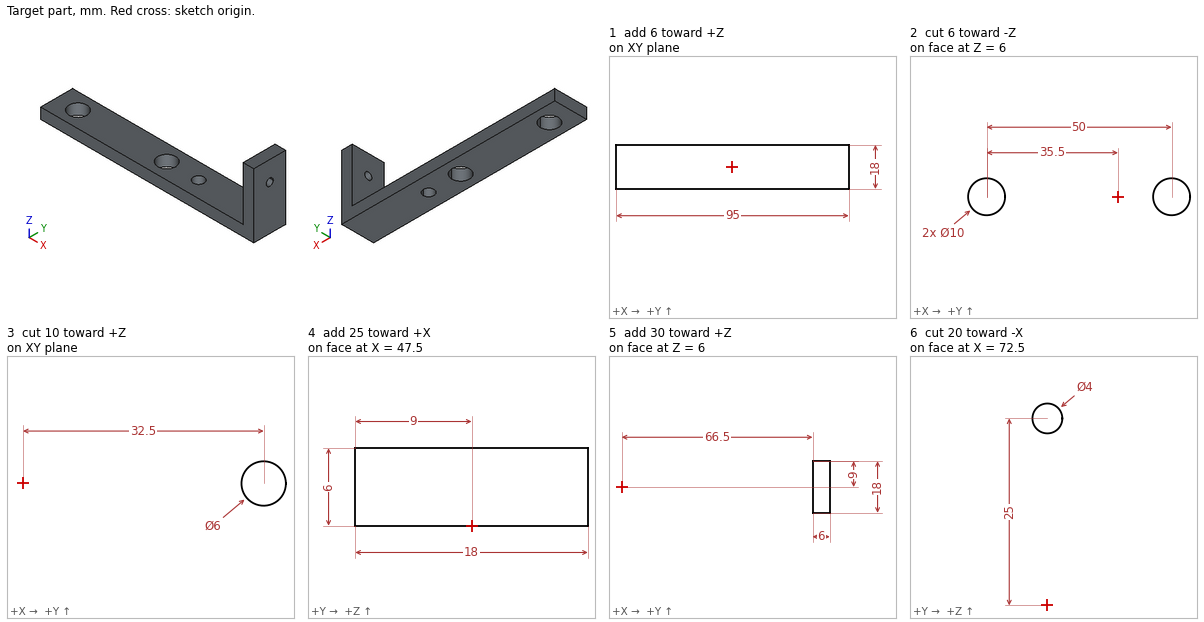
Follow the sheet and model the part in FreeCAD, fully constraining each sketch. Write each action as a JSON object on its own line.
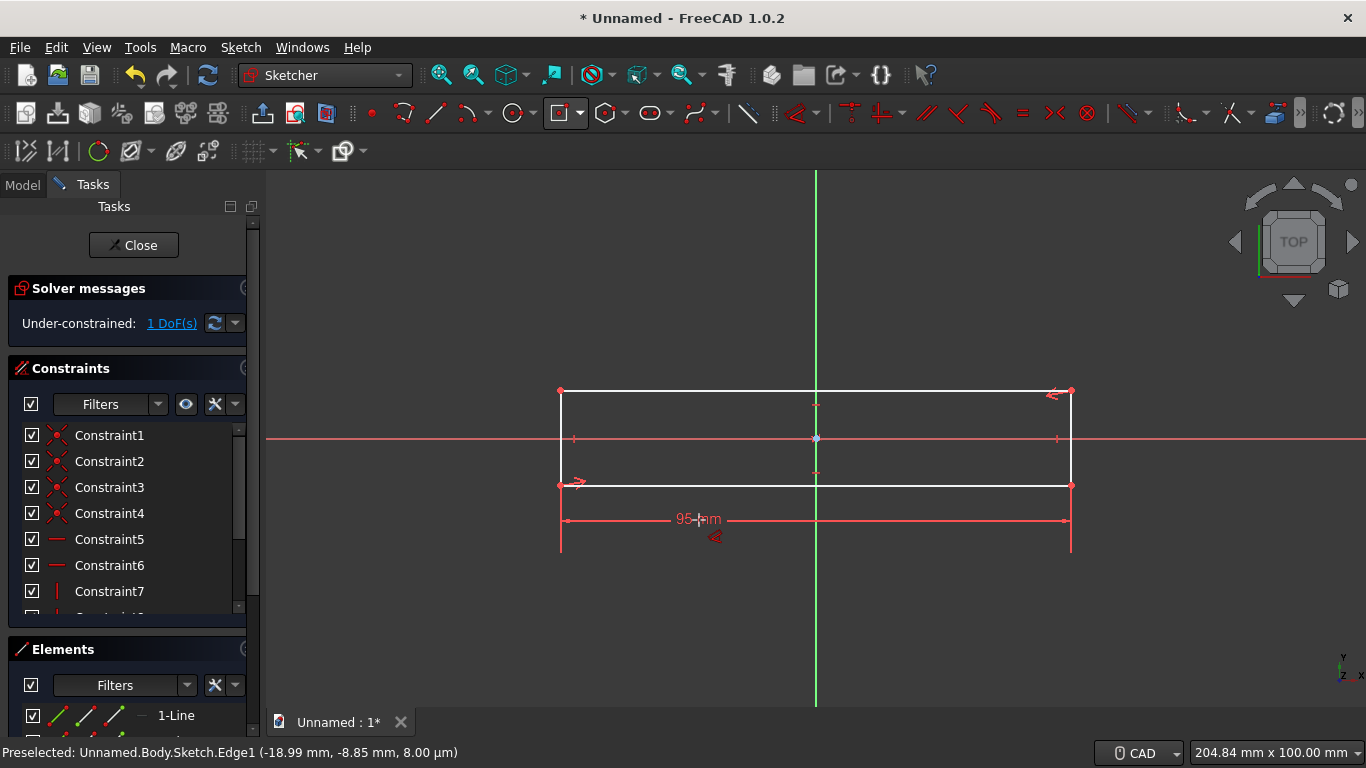
{"action": "left_click", "coordinate": [1071, 457]}
{"action": "left_click", "coordinate": [1105, 417]}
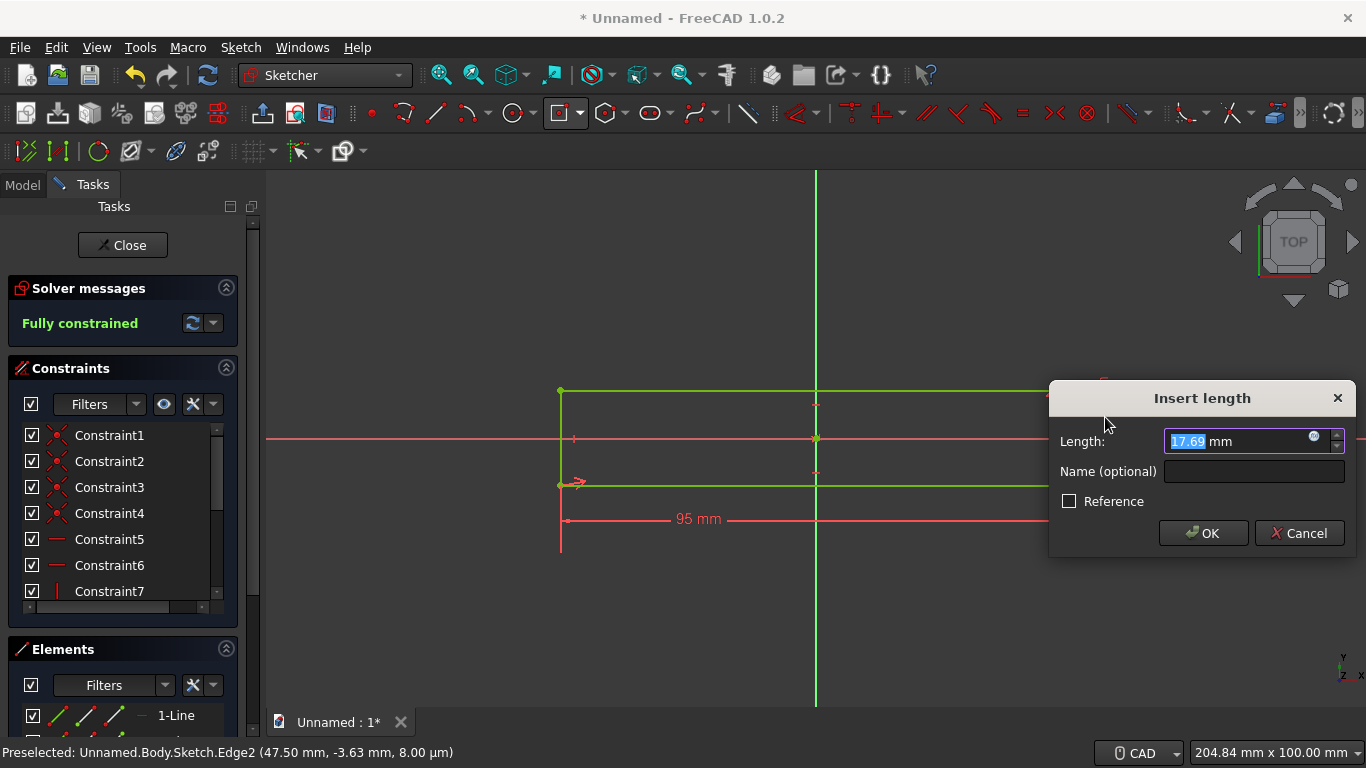
{"action": "type", "text": "18"}
{"action": "key", "text": "Return"}
{"action": "key", "text": "Escape"}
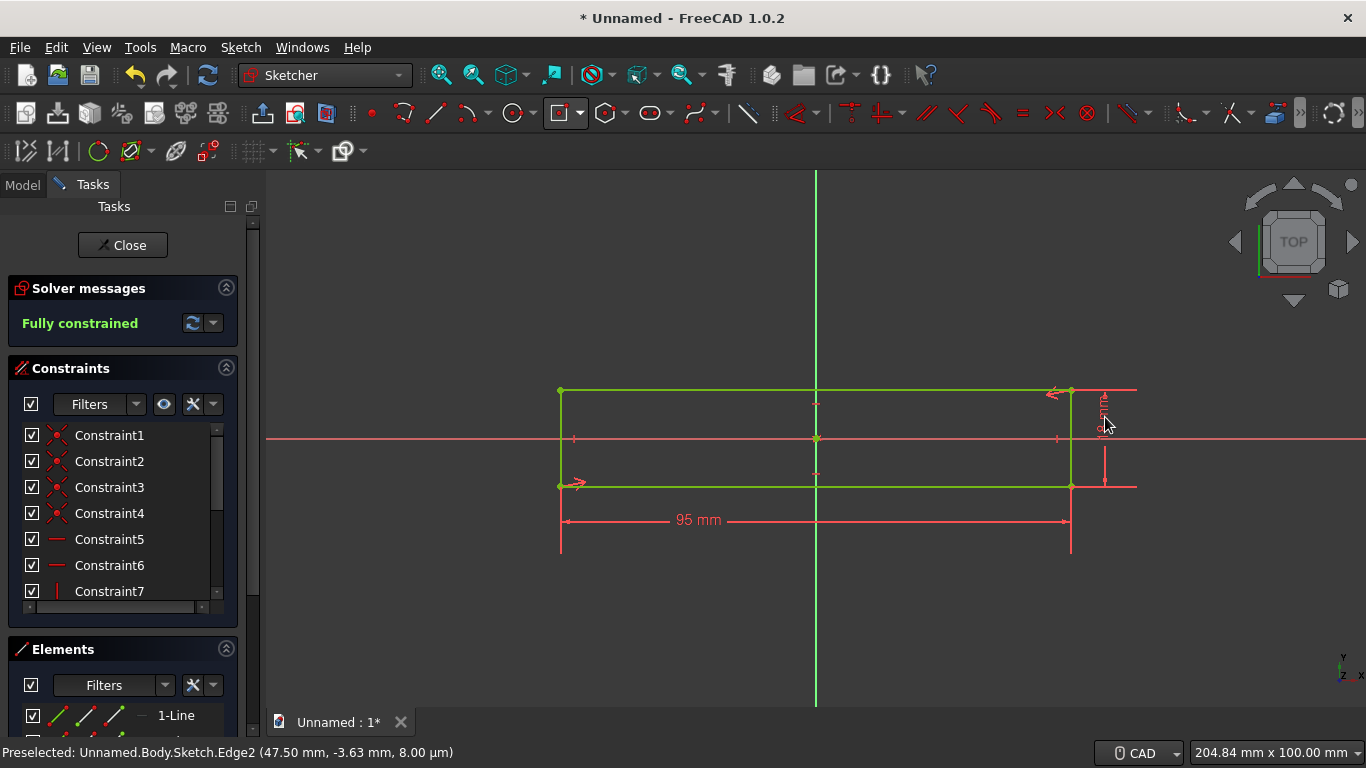
{"action": "left_click", "coordinate": [123, 245]}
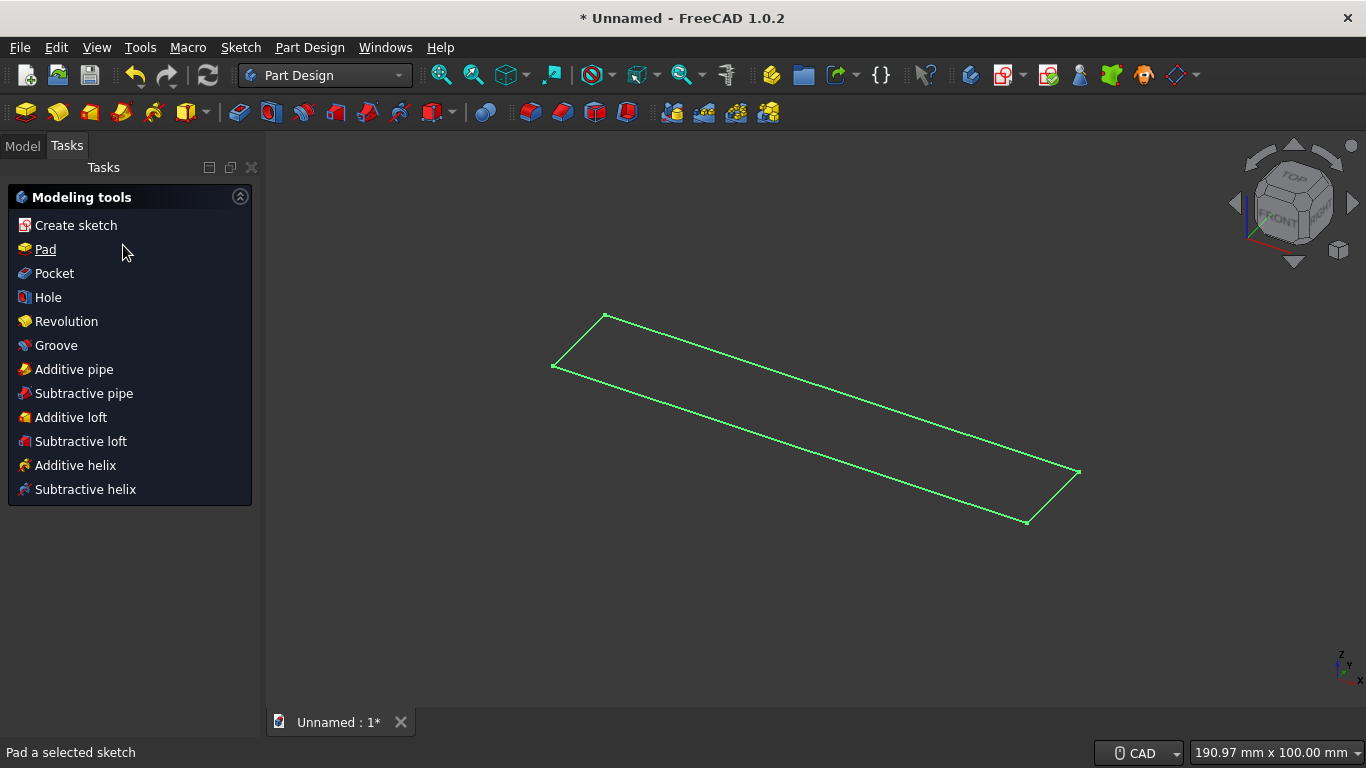
{"action": "left_click", "coordinate": [26, 112]}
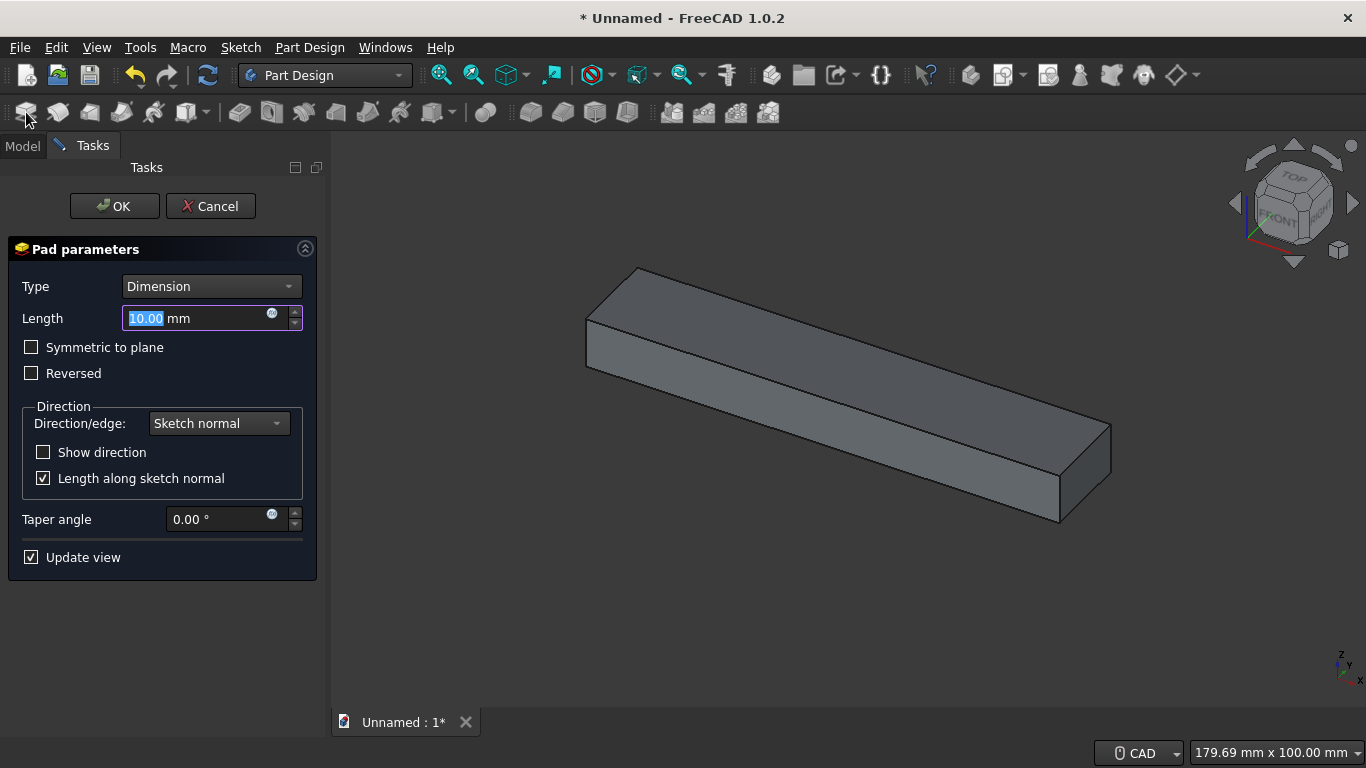
{"action": "type", "text": "6"}
{"action": "key", "text": "Tab"}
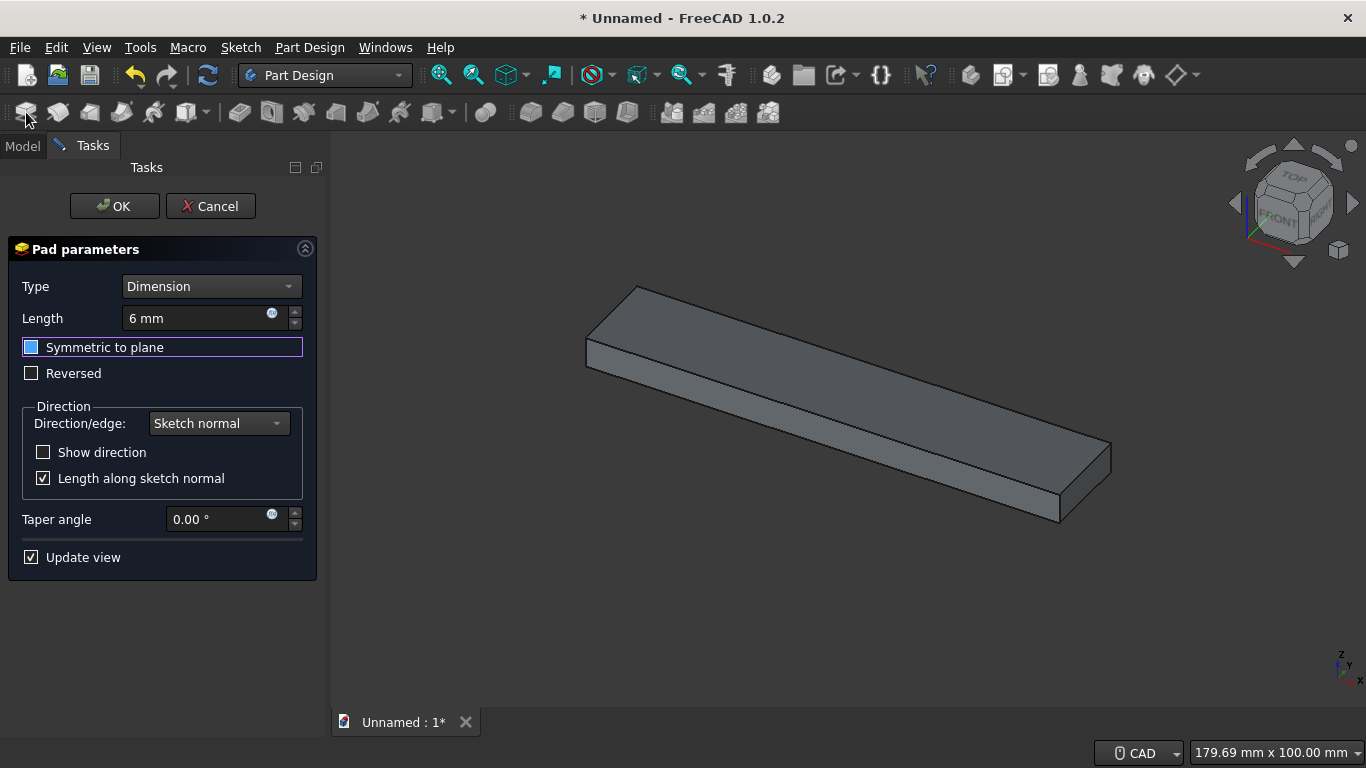
{"action": "left_click", "coordinate": [115, 206]}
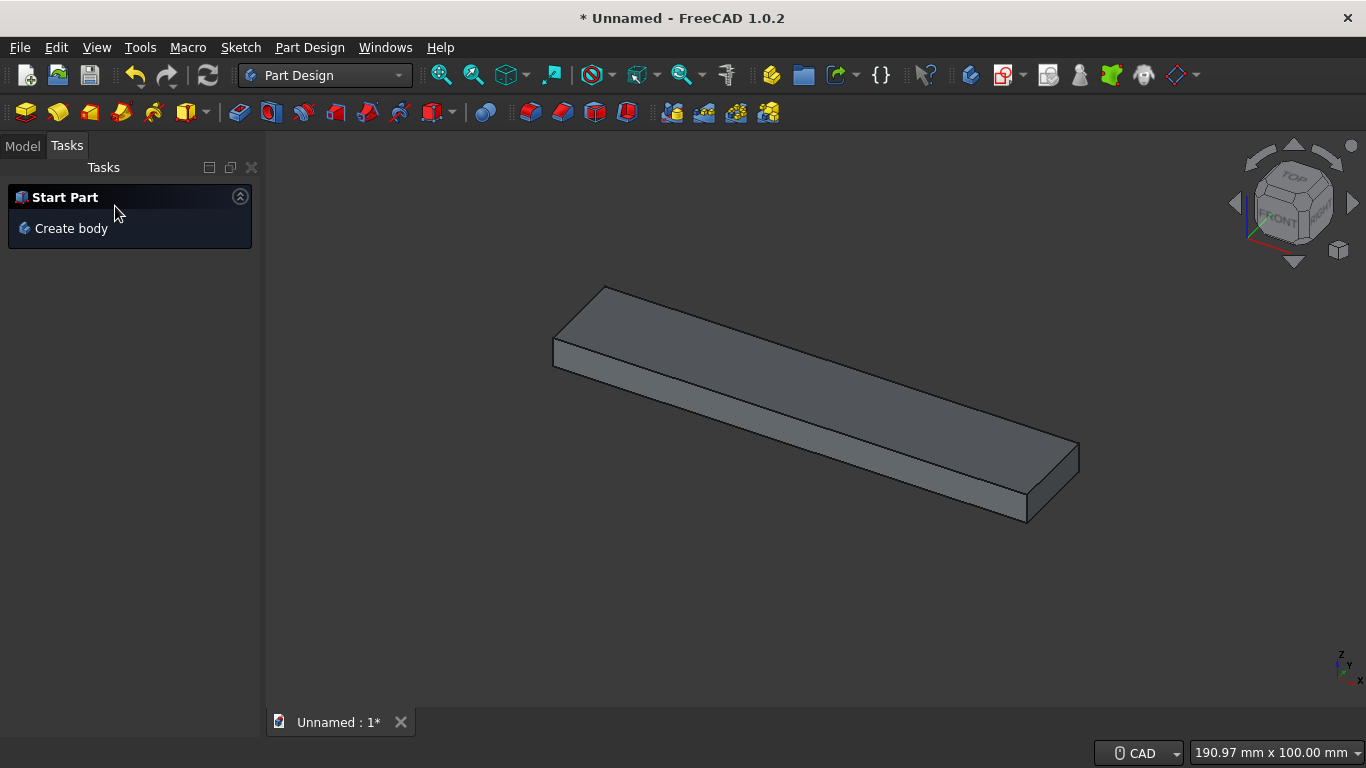
{"action": "left_click", "coordinate": [951, 435]}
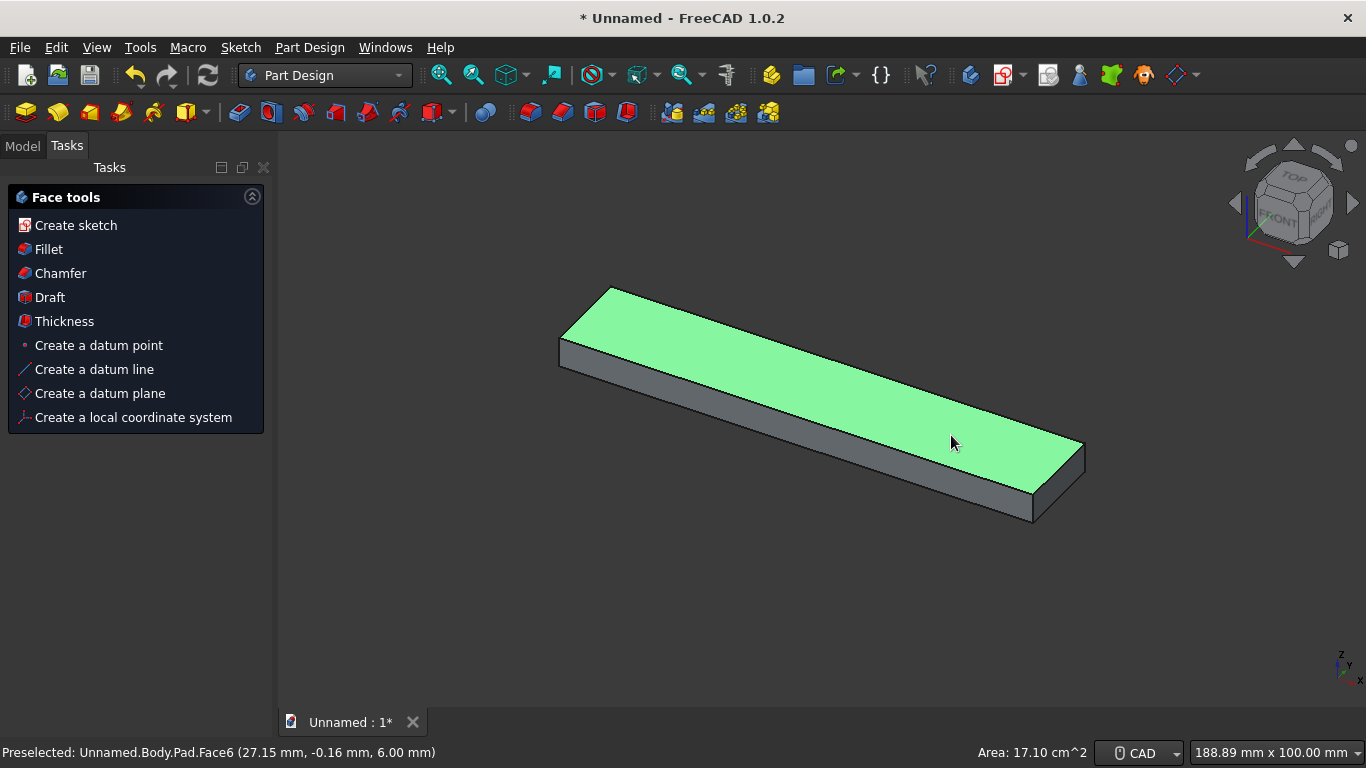
{"action": "left_click", "coordinate": [1004, 76]}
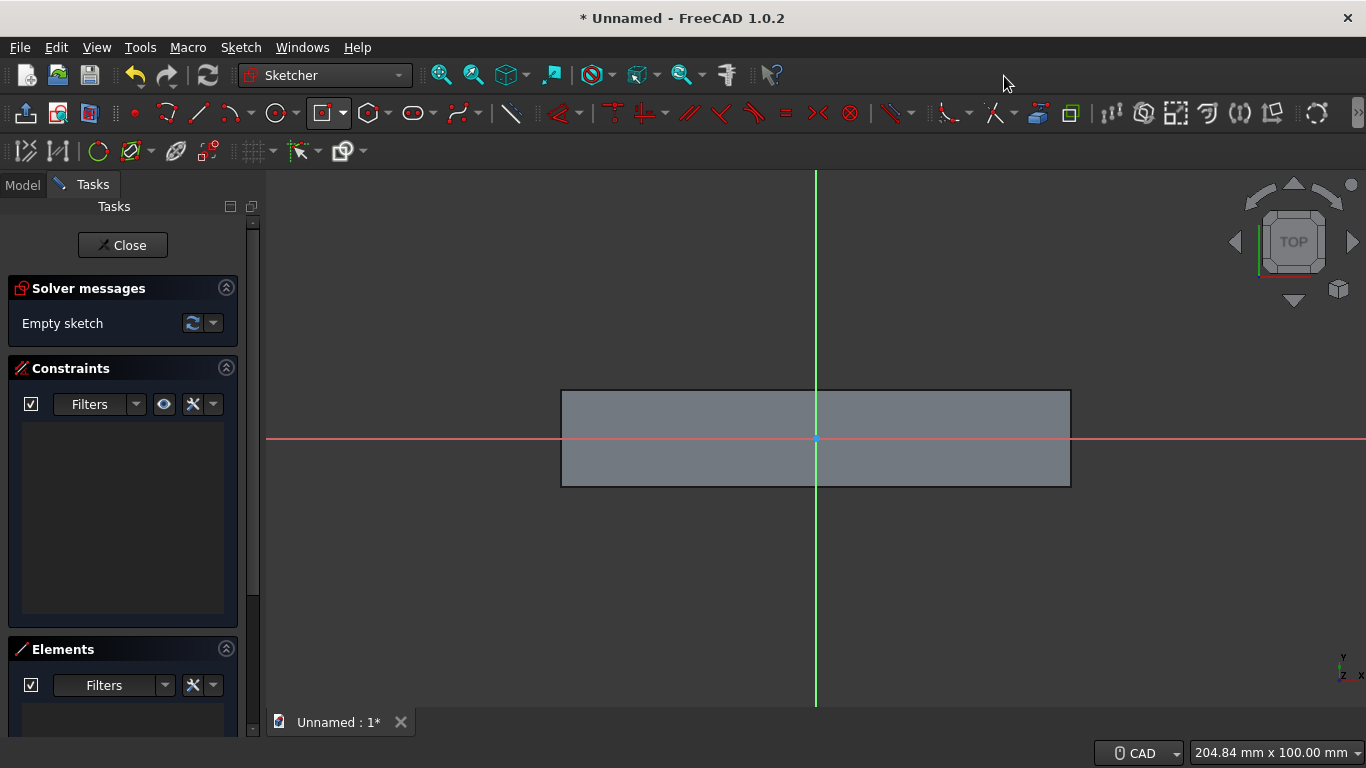
{"action": "scroll", "coordinate": [774, 438], "scroll_direction": "up", "scroll_amount": 3}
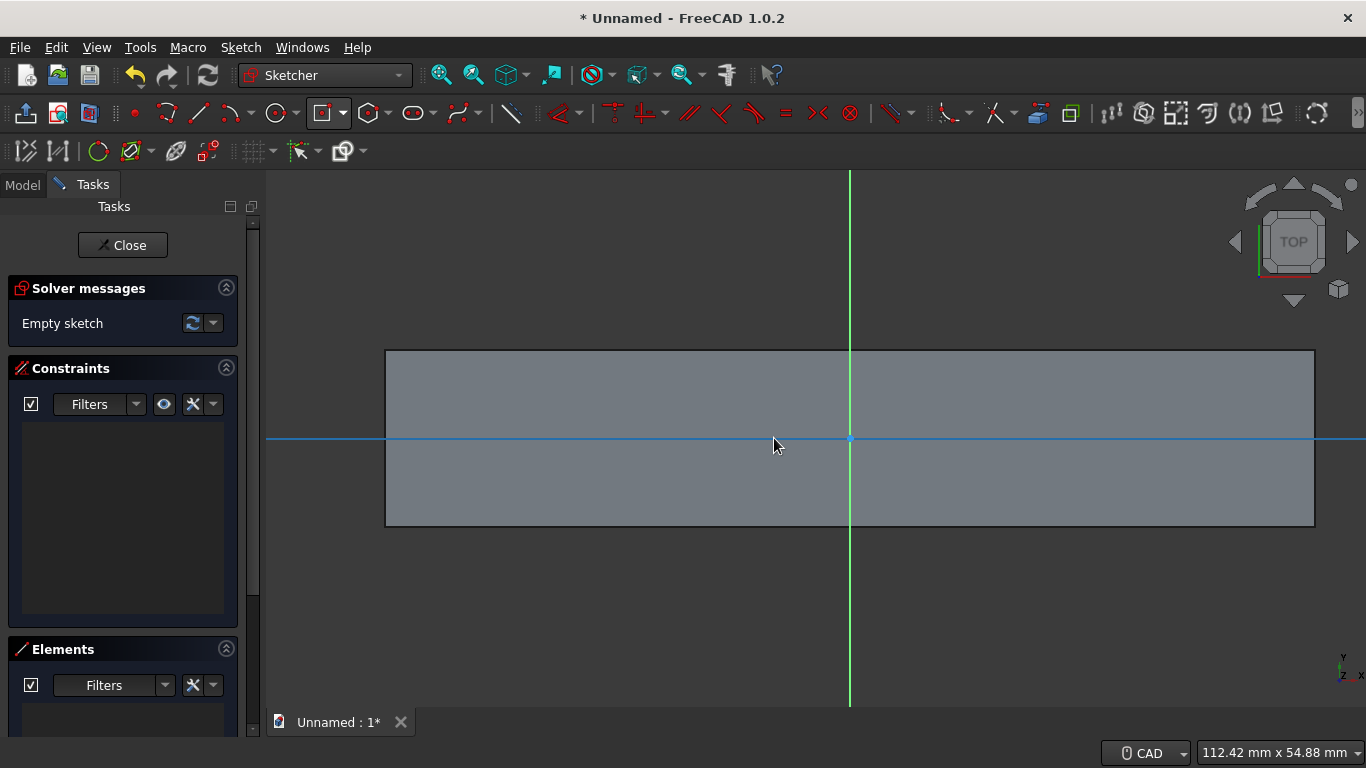
{"action": "left_click", "coordinate": [276, 114]}